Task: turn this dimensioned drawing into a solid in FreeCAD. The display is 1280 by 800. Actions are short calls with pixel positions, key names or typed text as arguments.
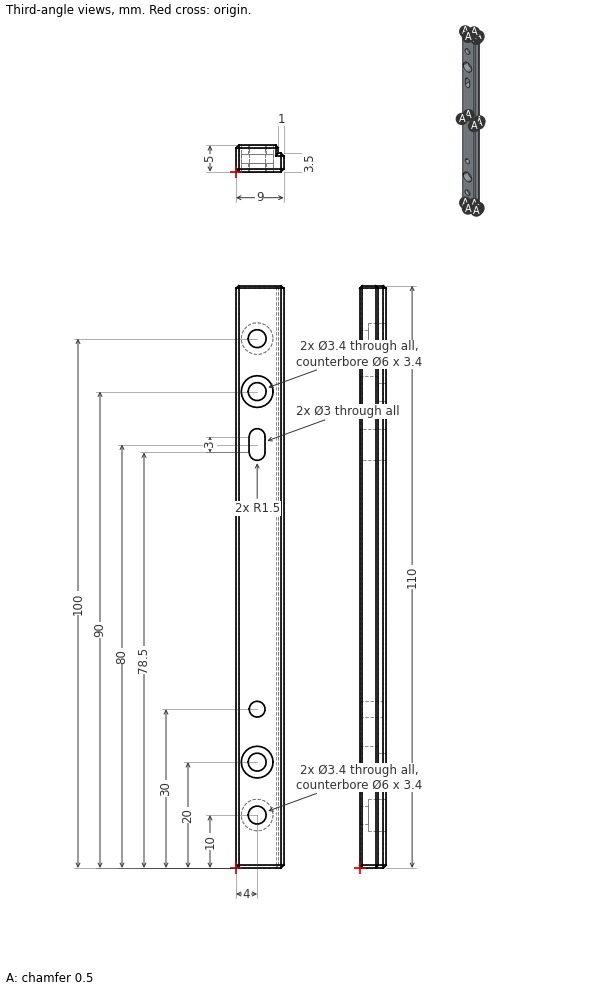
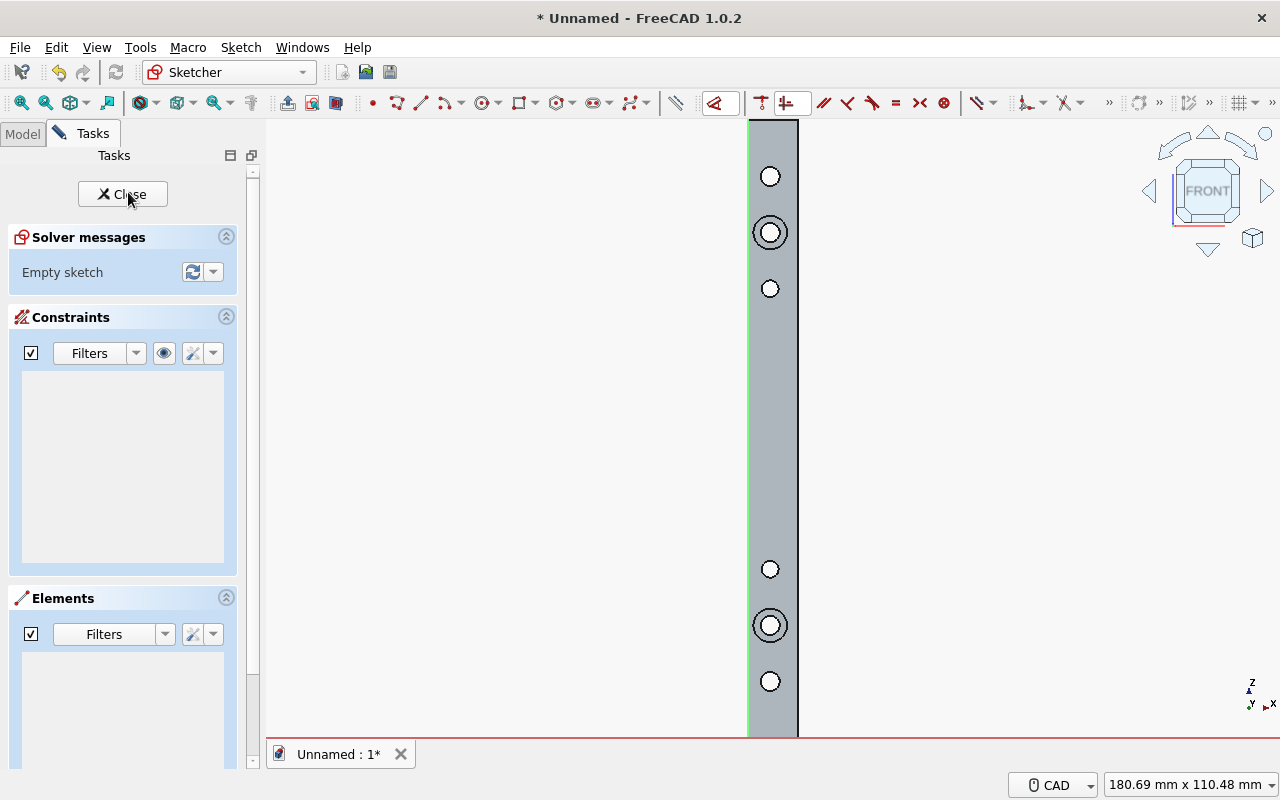
scroll(777, 275, up, 12)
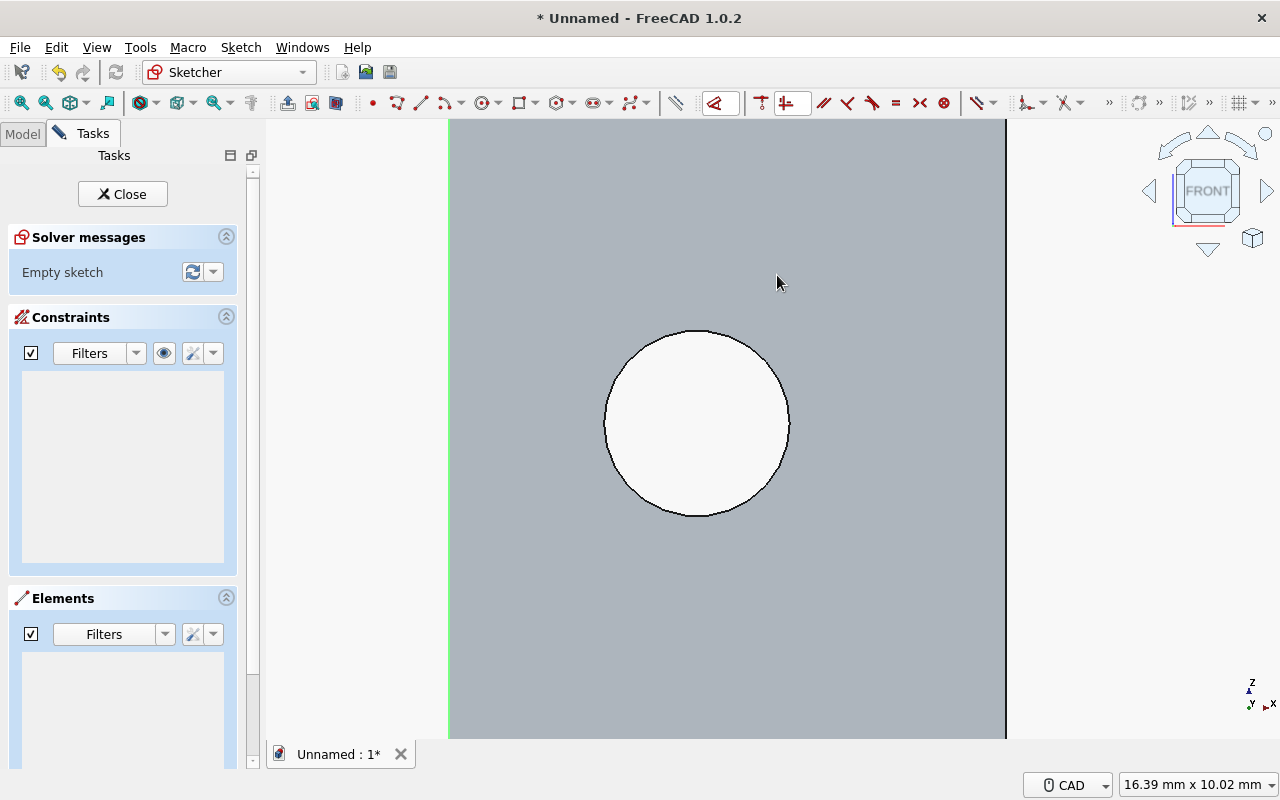
key(g)
key(s)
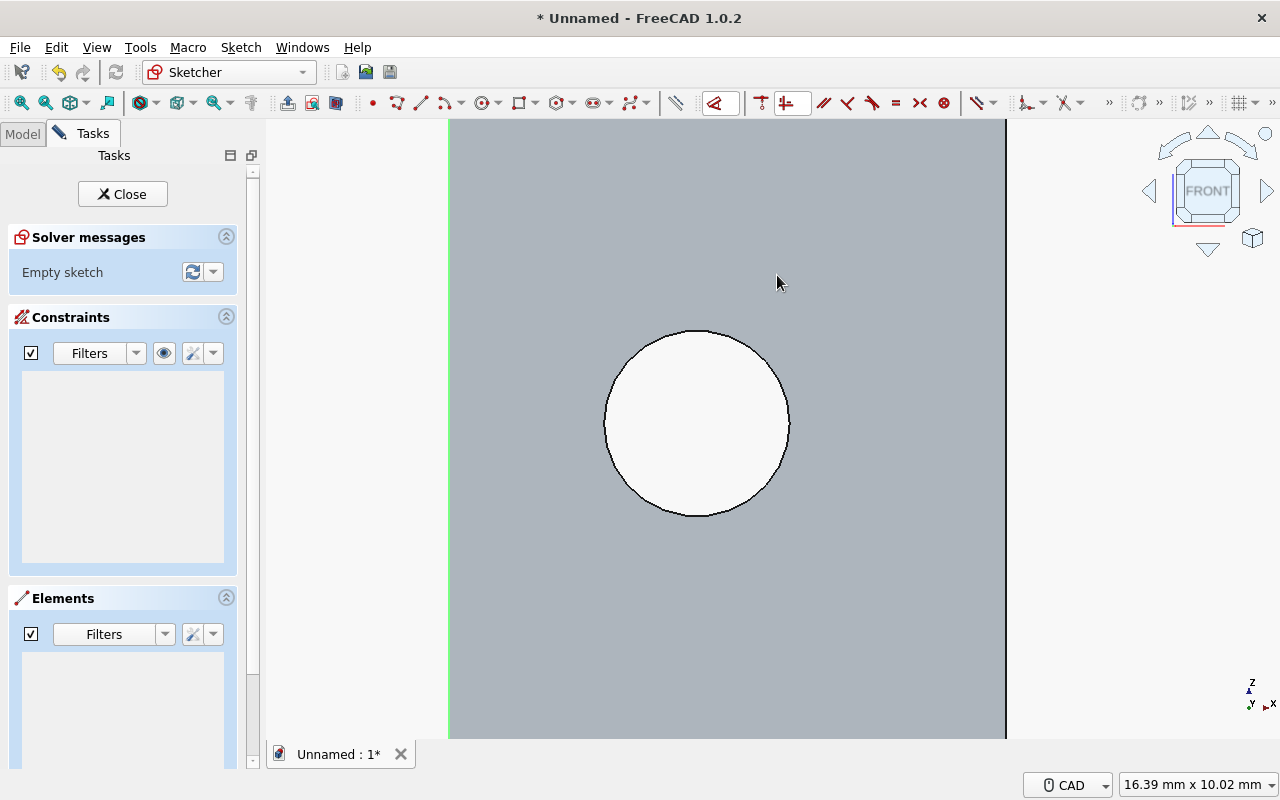
click(697, 516)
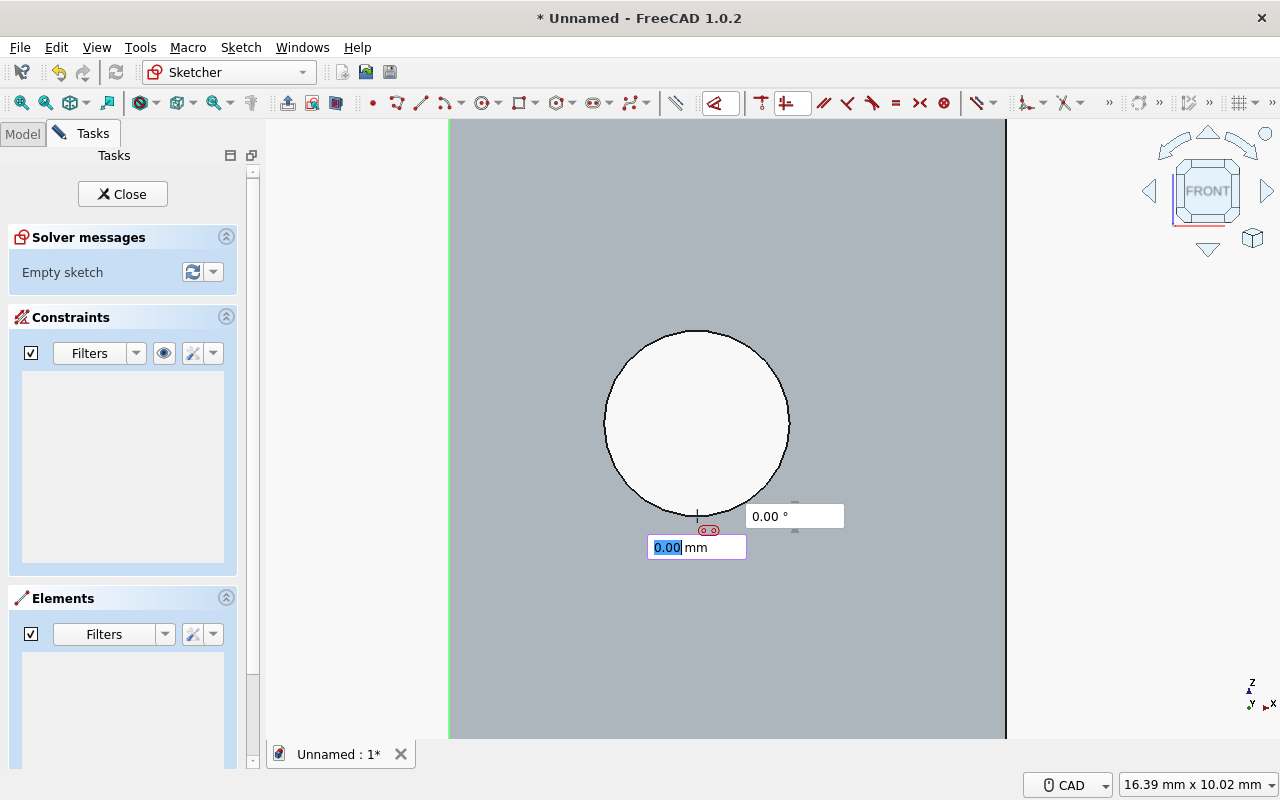
click(697, 331)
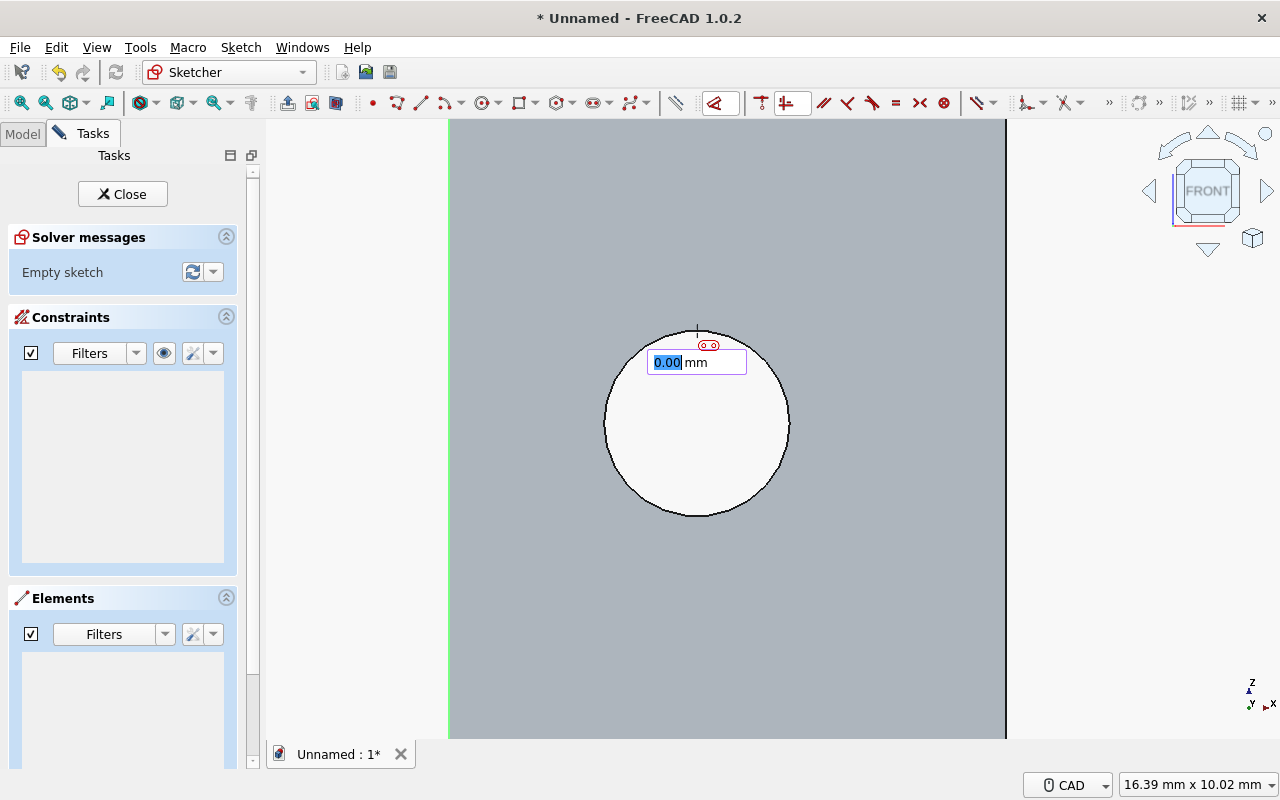
click(604, 424)
key(Escape)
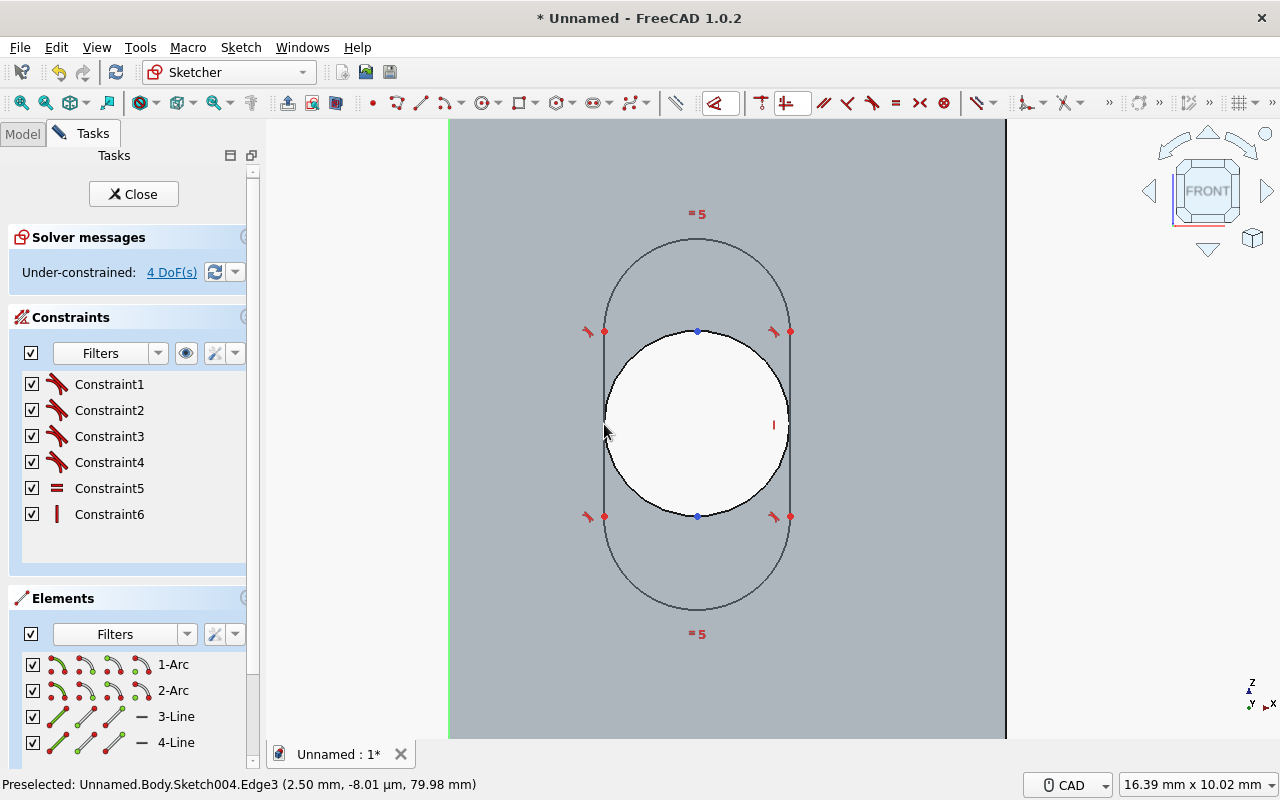
key(d)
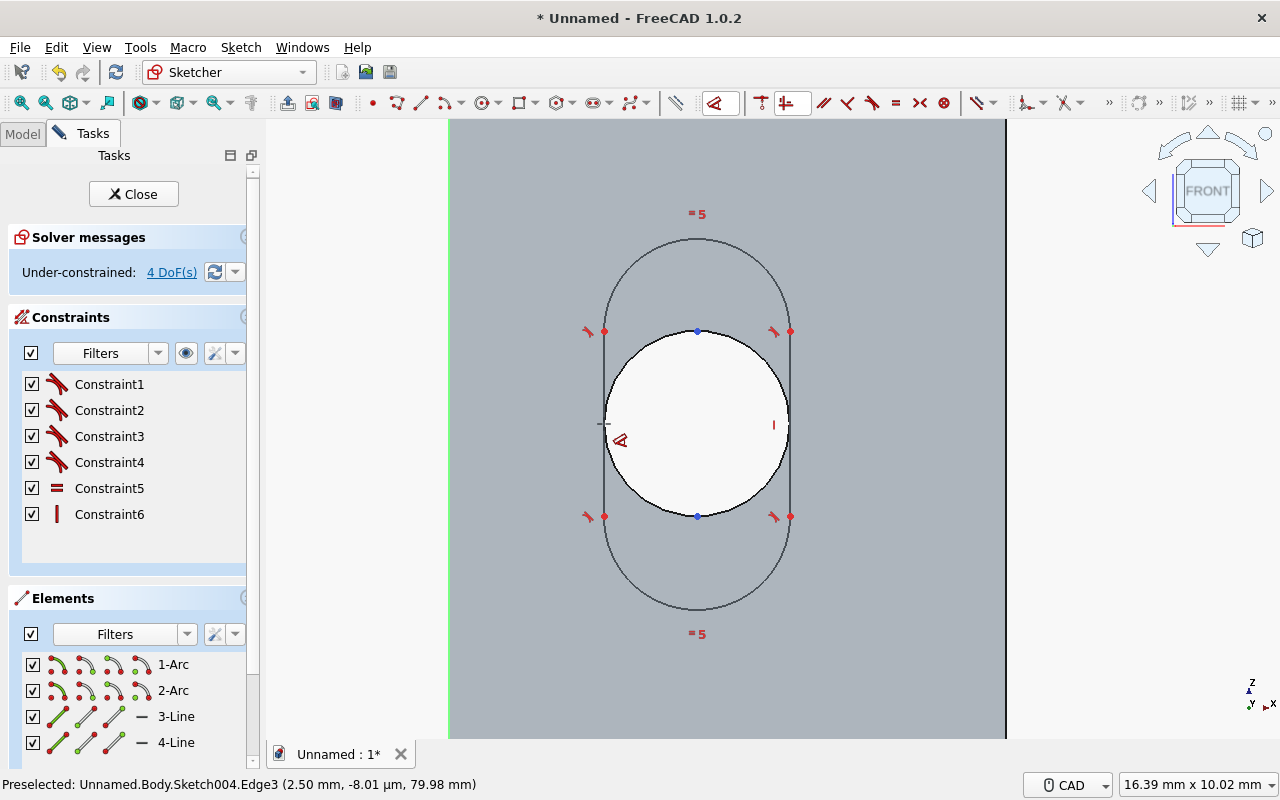
click(642, 592)
click(623, 618)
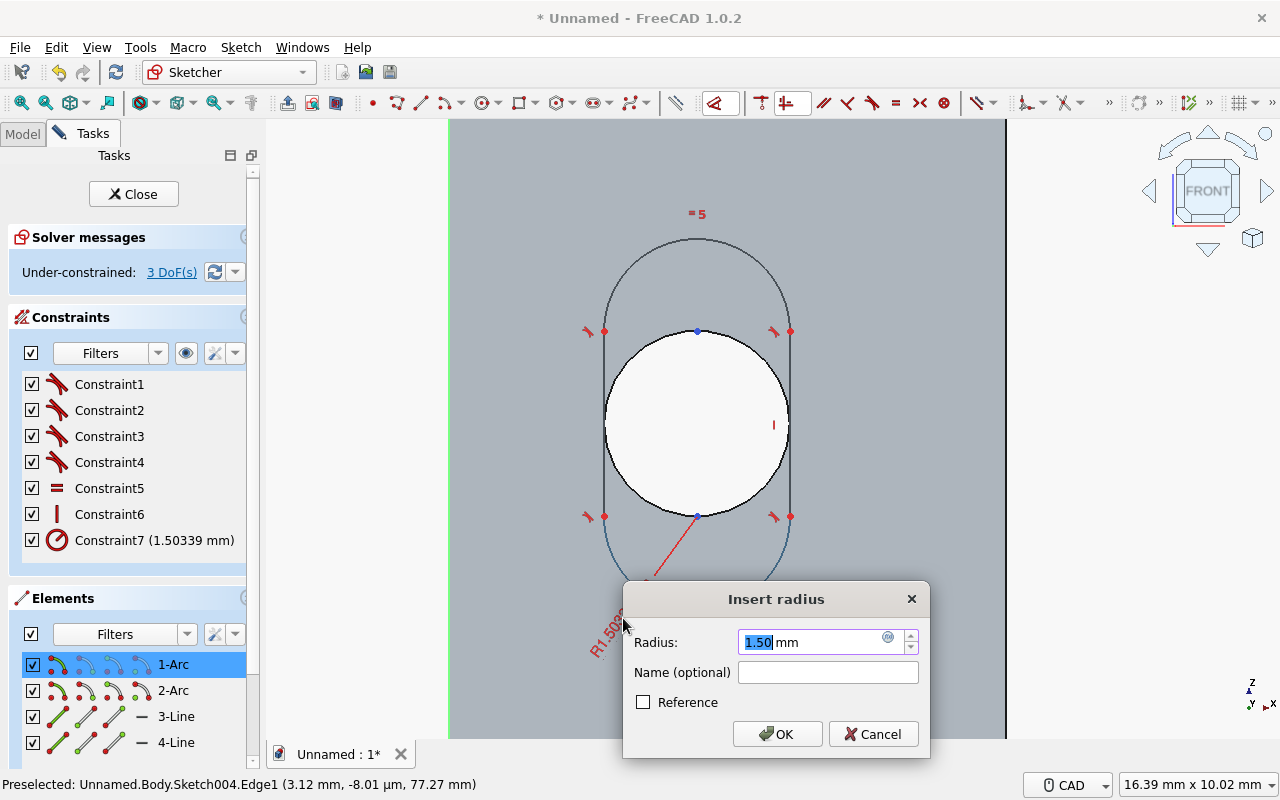
text(1.5)
key(Return)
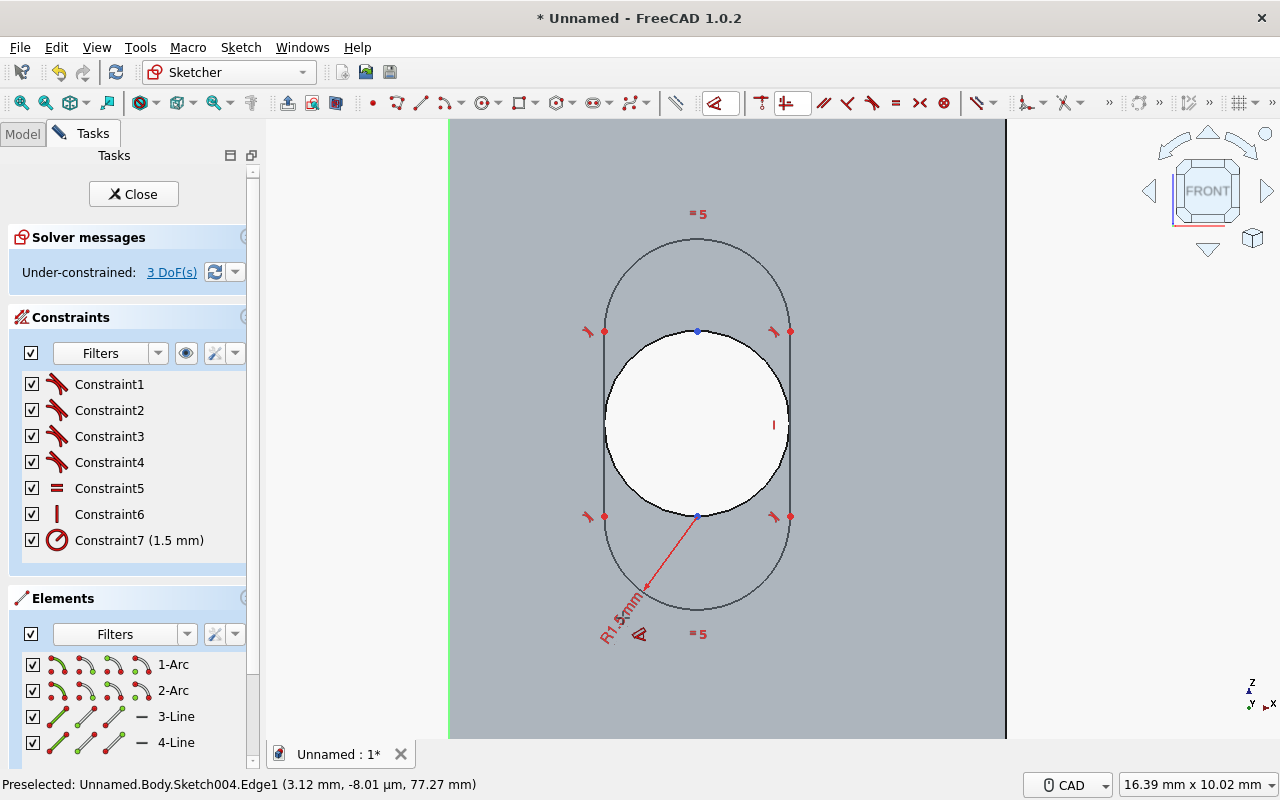
click(604, 461)
click(570, 424)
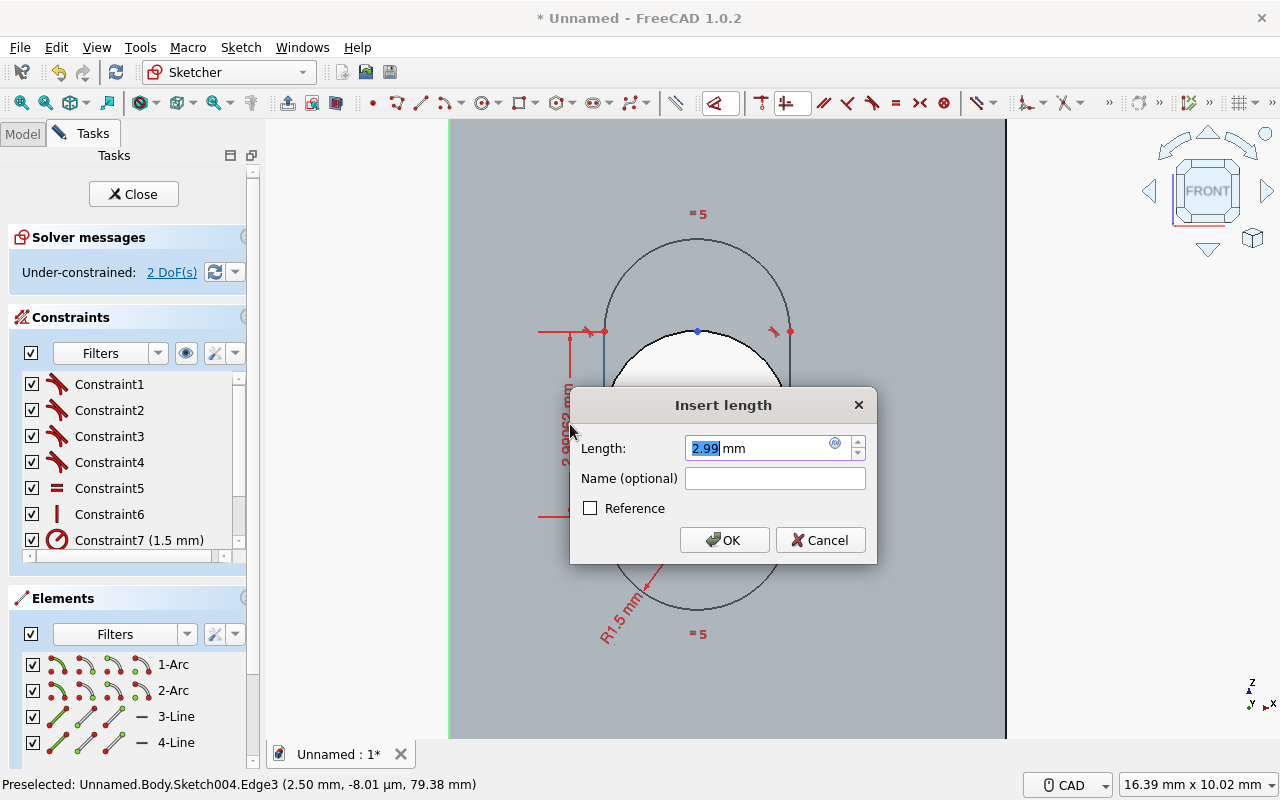
text(3)
key(Return)